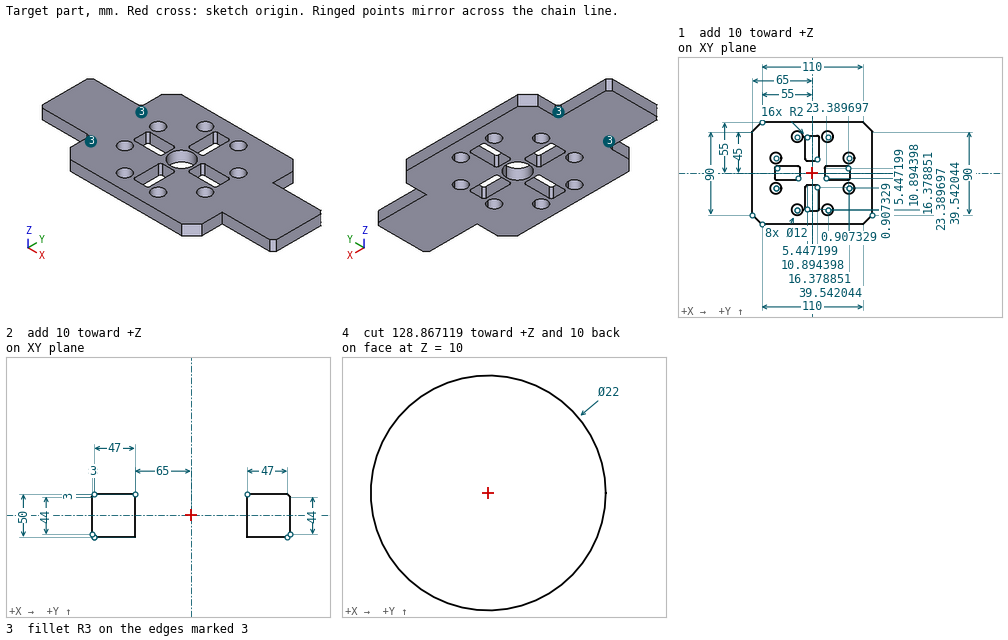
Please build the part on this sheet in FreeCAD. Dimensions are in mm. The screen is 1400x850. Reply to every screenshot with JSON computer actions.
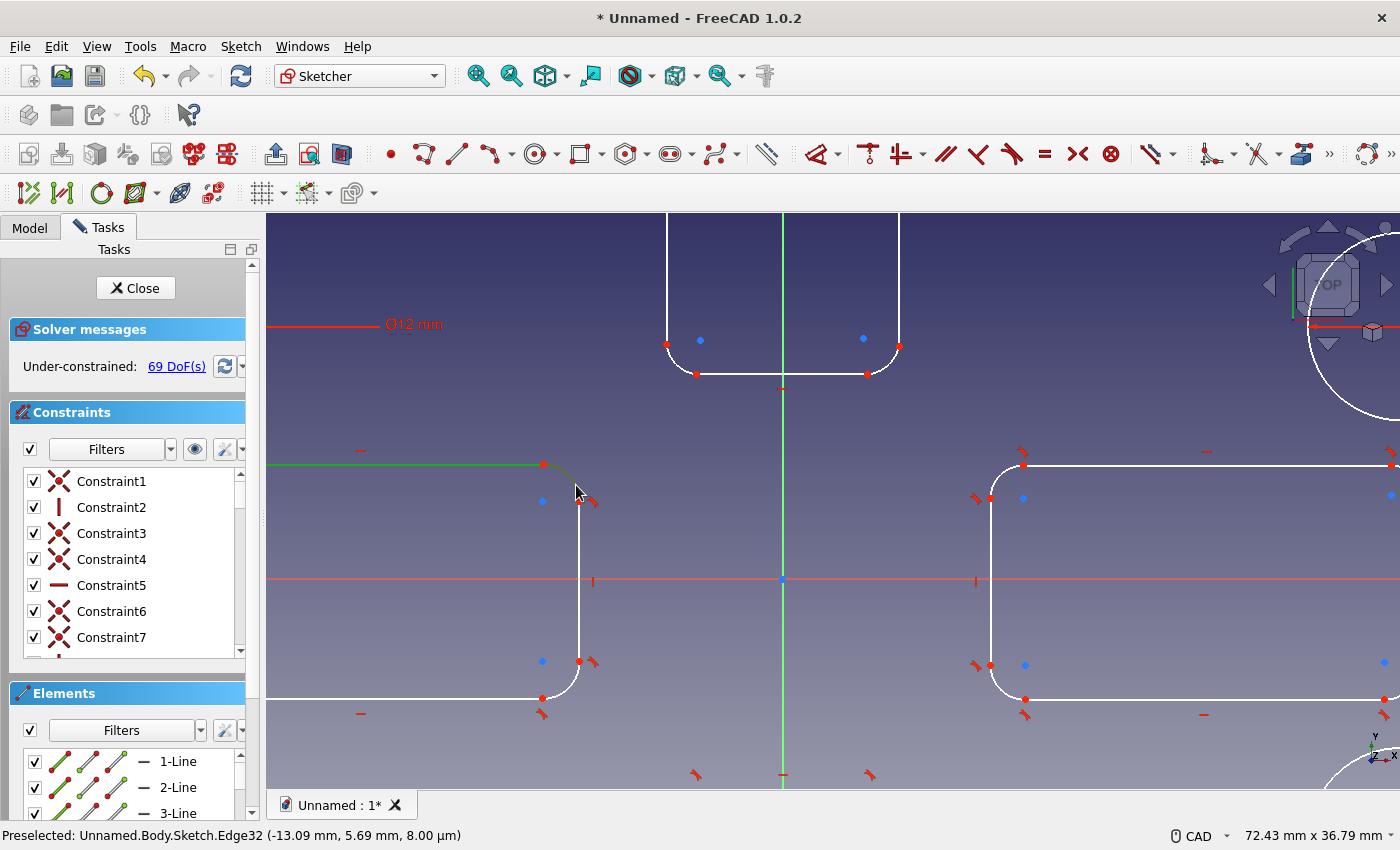
{"action": "left_click", "coordinate": [1012, 154]}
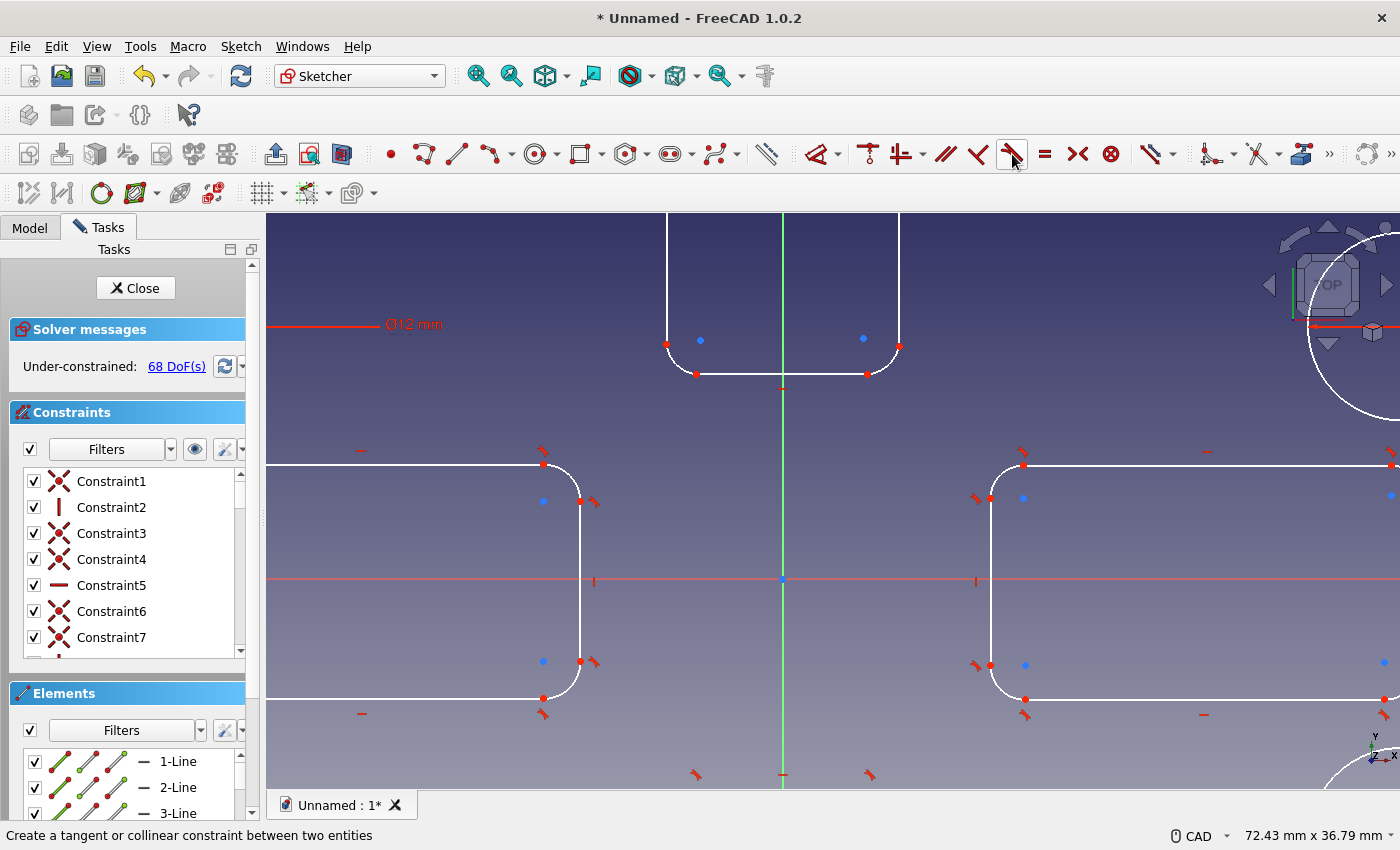
{"action": "scroll", "coordinate": [760, 481], "scroll_direction": "down", "scroll_amount": 8}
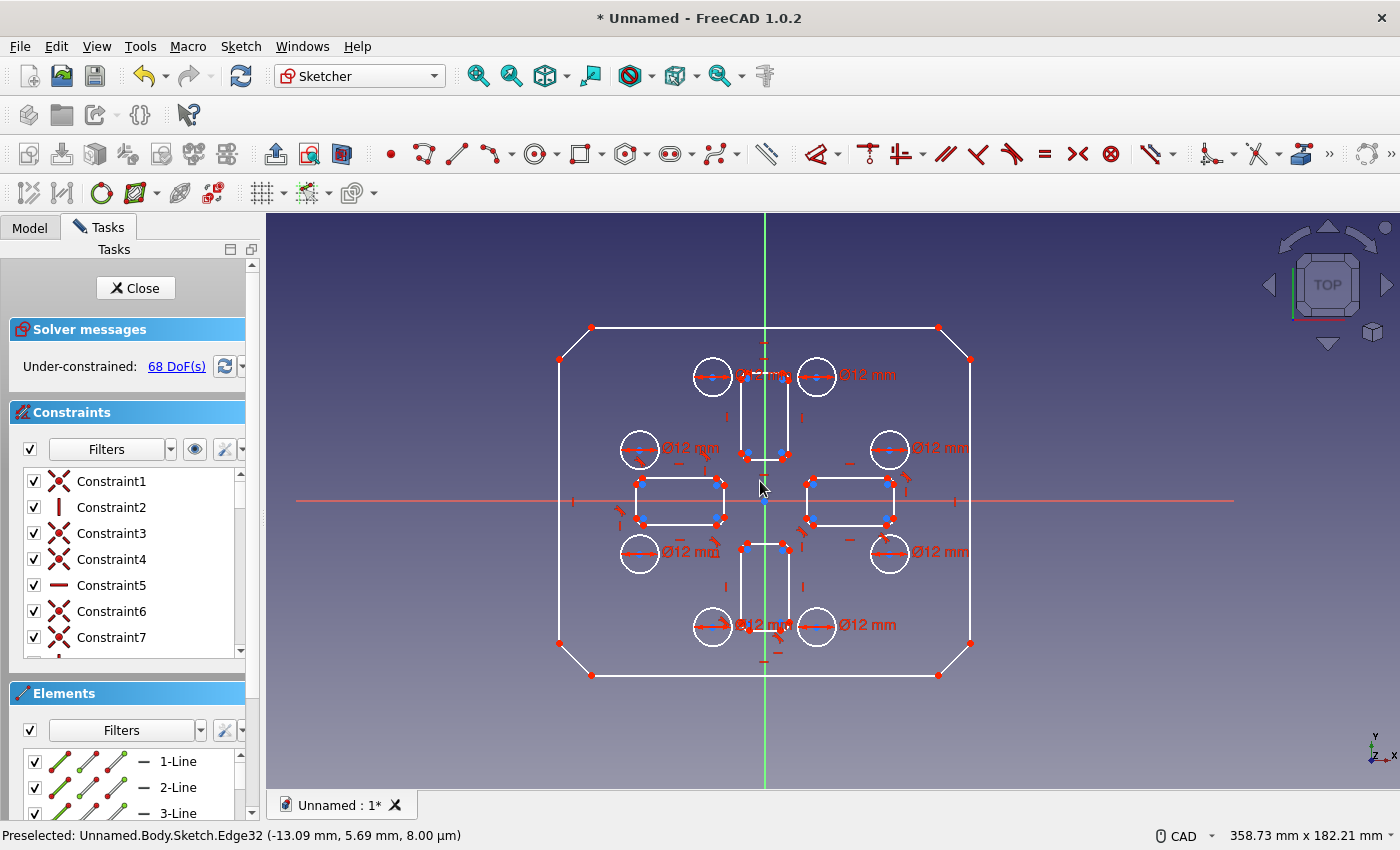
{"action": "left_click", "coordinate": [788, 439]}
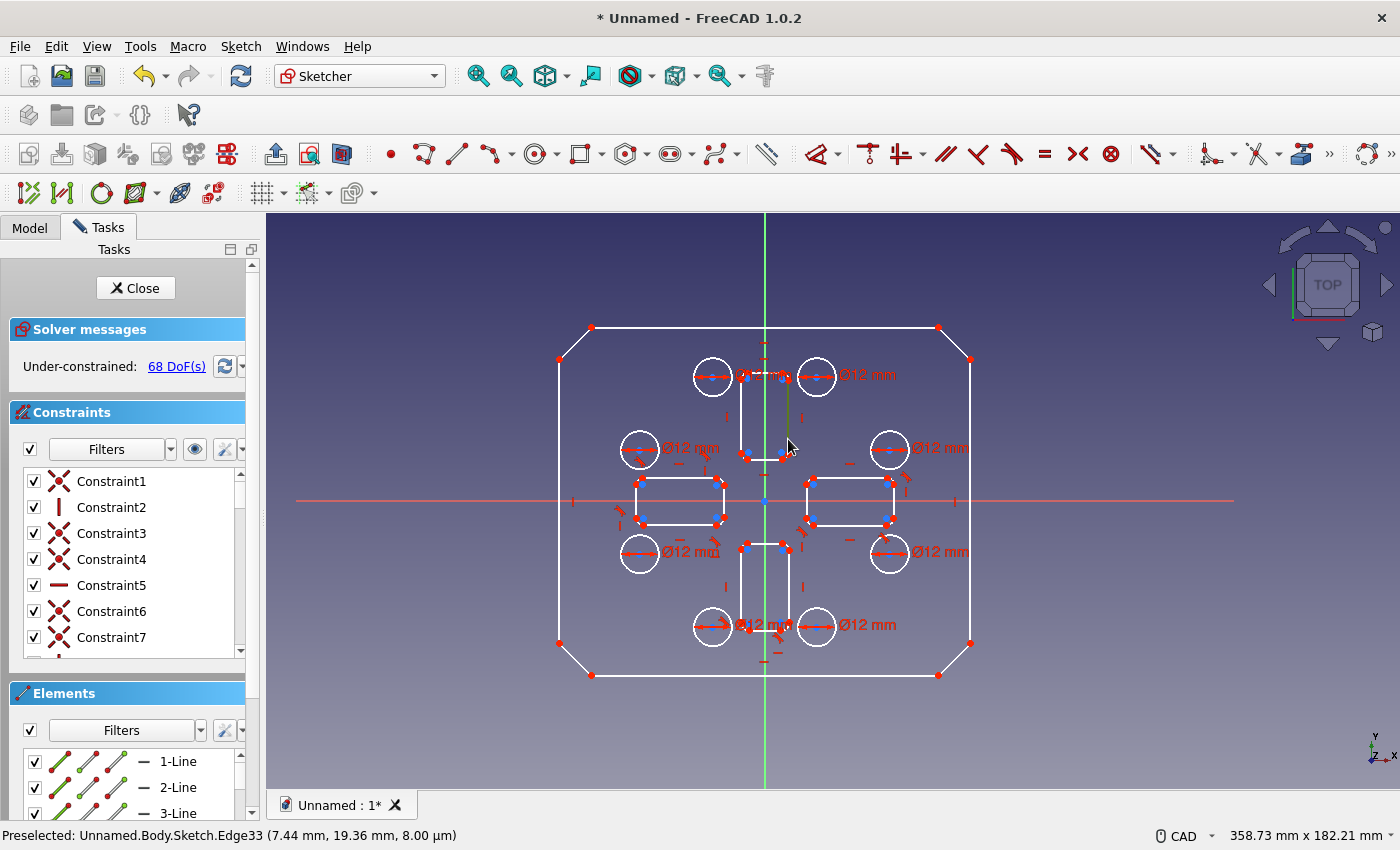
{"action": "scroll", "coordinate": [786, 458], "scroll_direction": "up", "scroll_amount": 6}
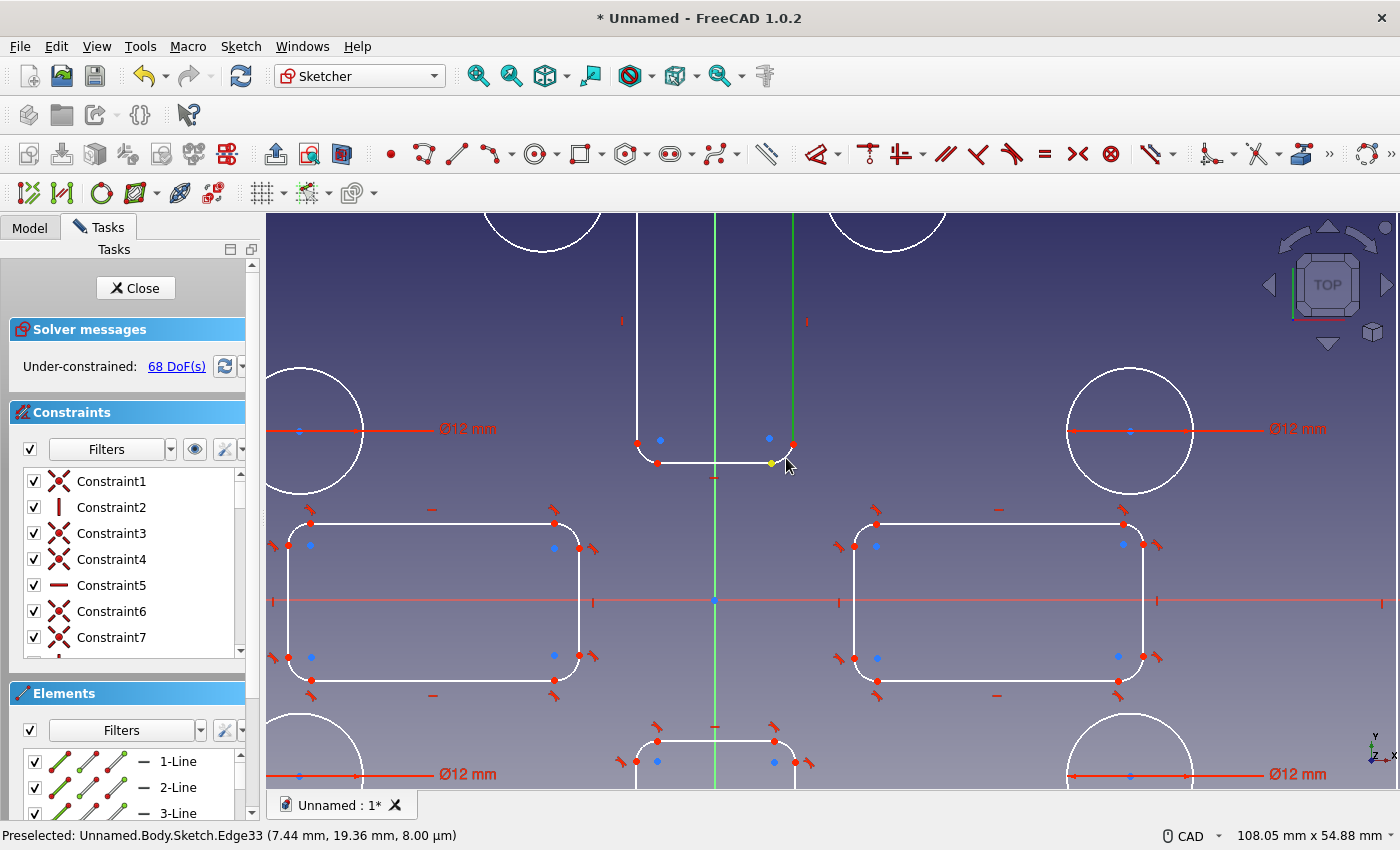
{"action": "left_click", "coordinate": [786, 457]}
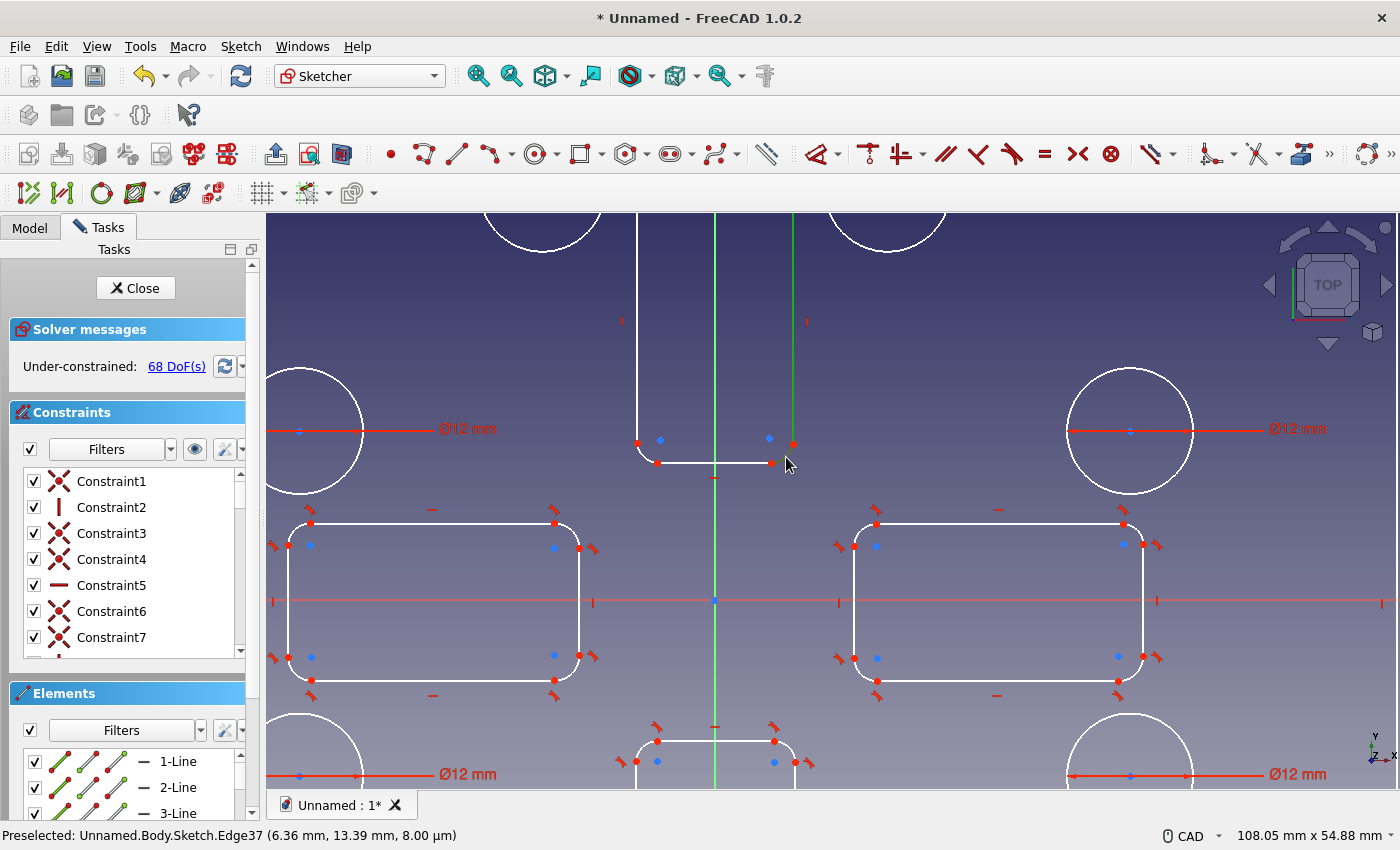
{"action": "left_click", "coordinate": [1012, 154]}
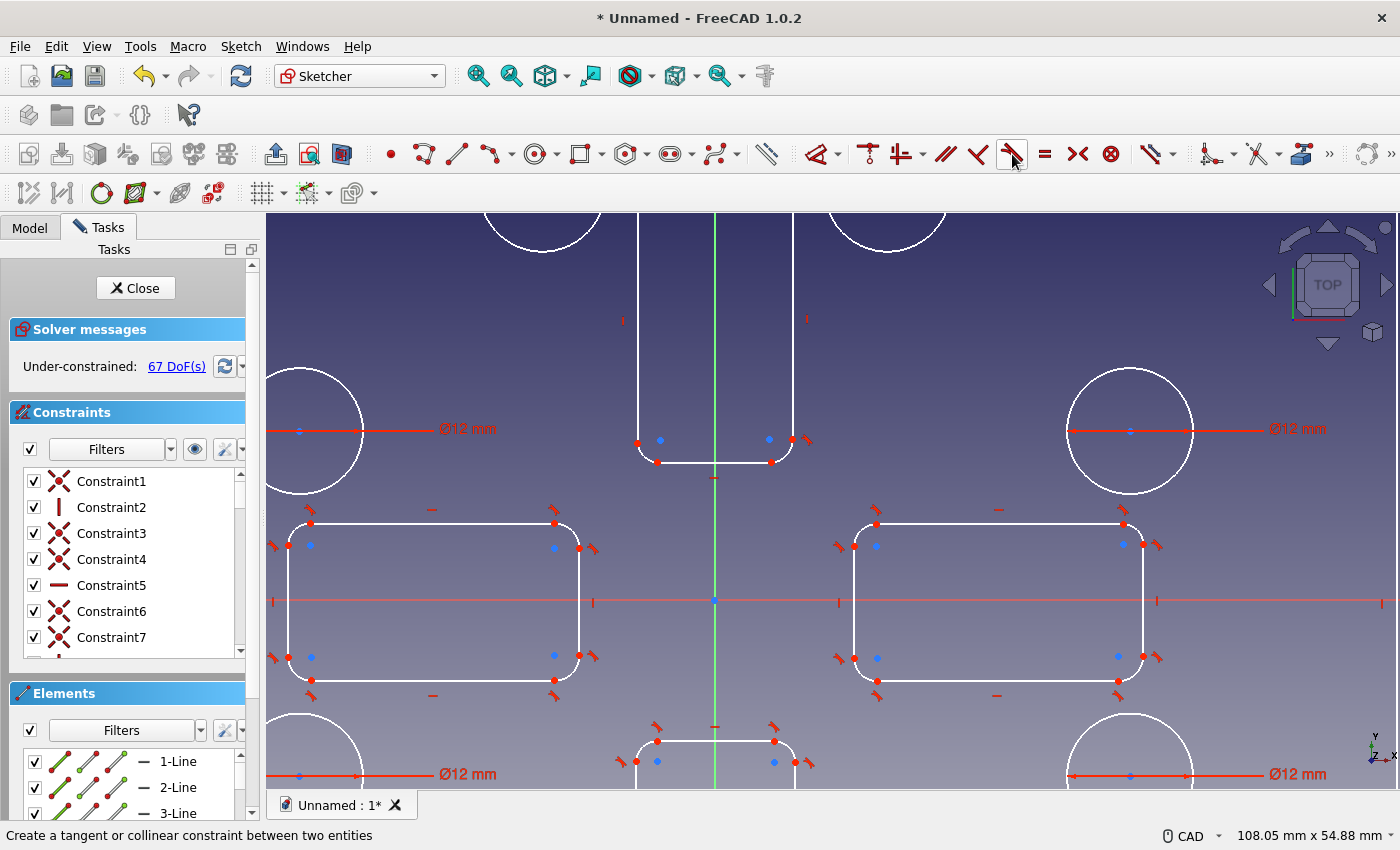
{"action": "left_click", "coordinate": [793, 271]}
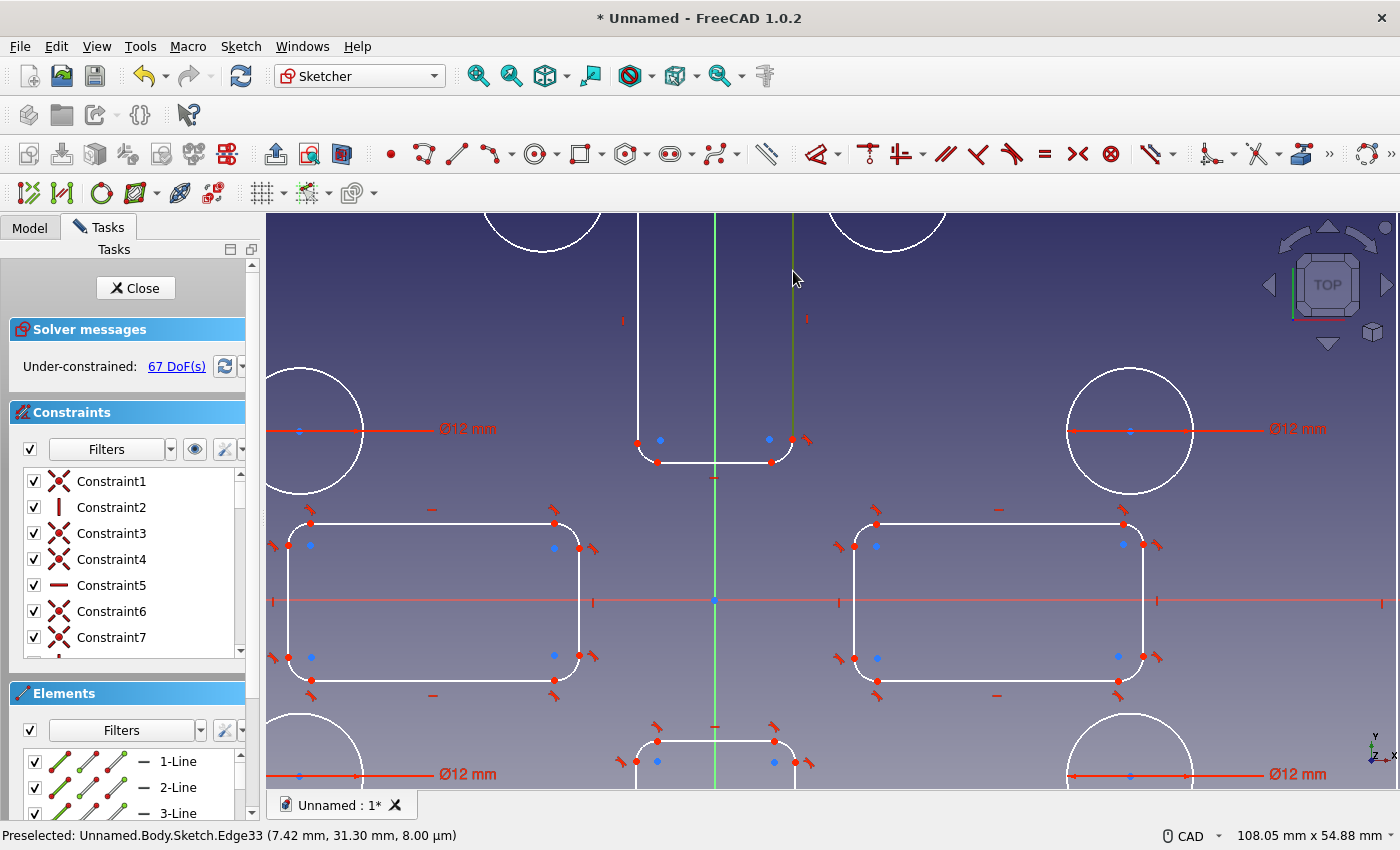
{"action": "scroll", "coordinate": [786, 458], "scroll_direction": "down", "scroll_amount": 6}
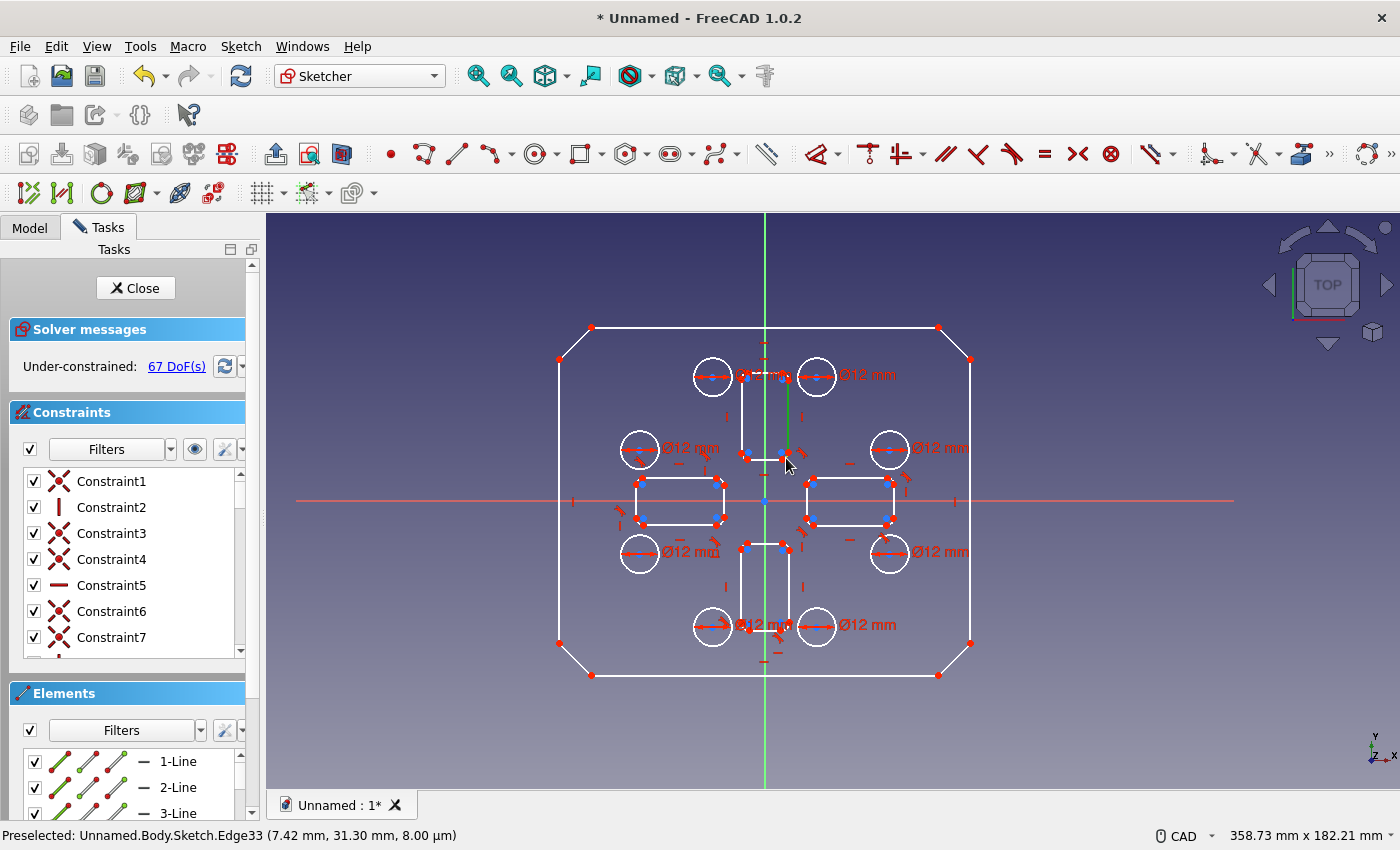
{"action": "scroll", "coordinate": [788, 377], "scroll_direction": "up", "scroll_amount": 8}